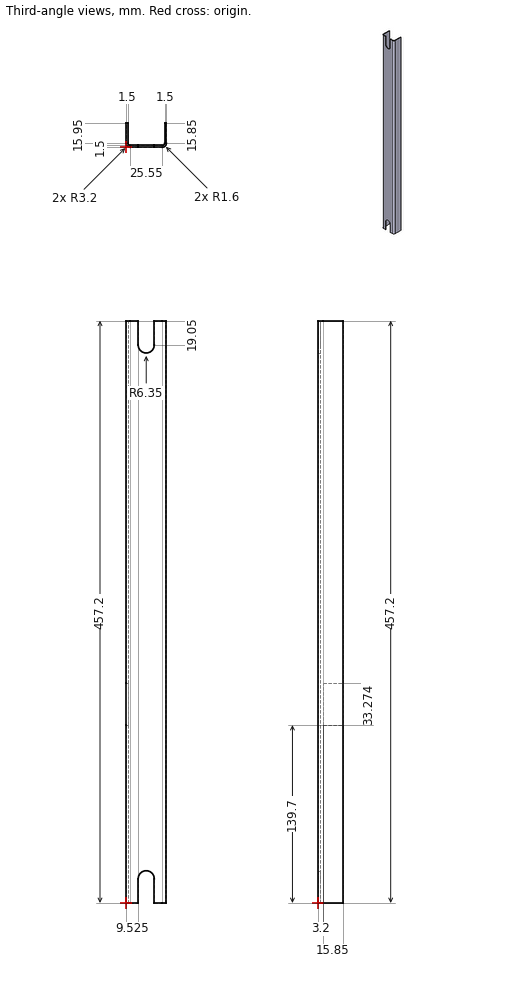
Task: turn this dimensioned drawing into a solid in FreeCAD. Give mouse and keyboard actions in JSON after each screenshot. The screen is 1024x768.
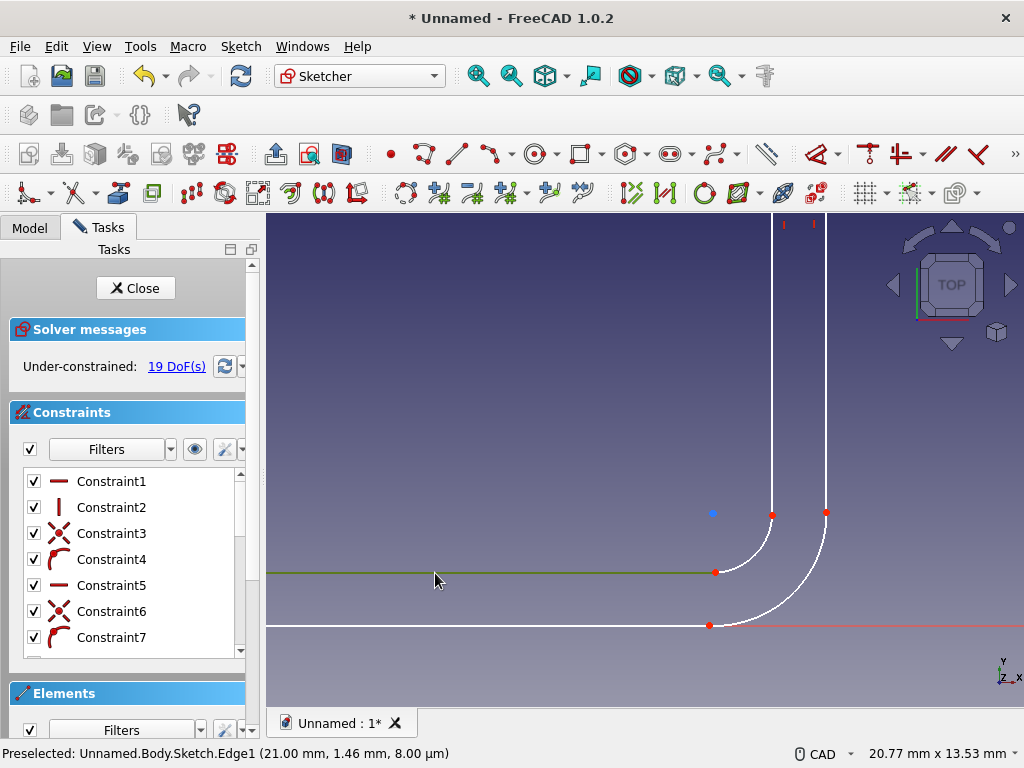
{"action": "scroll", "coordinate": [768, 566], "scroll_direction": "down", "scroll_amount": 5}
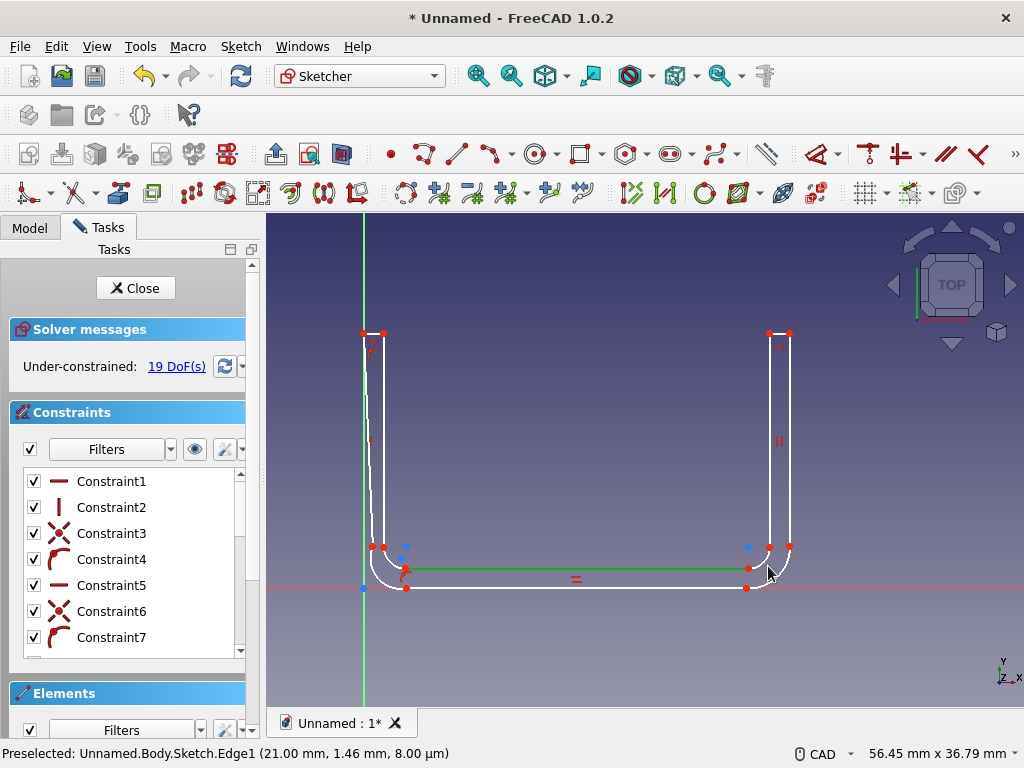
{"action": "scroll", "coordinate": [387, 557], "scroll_direction": "up", "scroll_amount": 2}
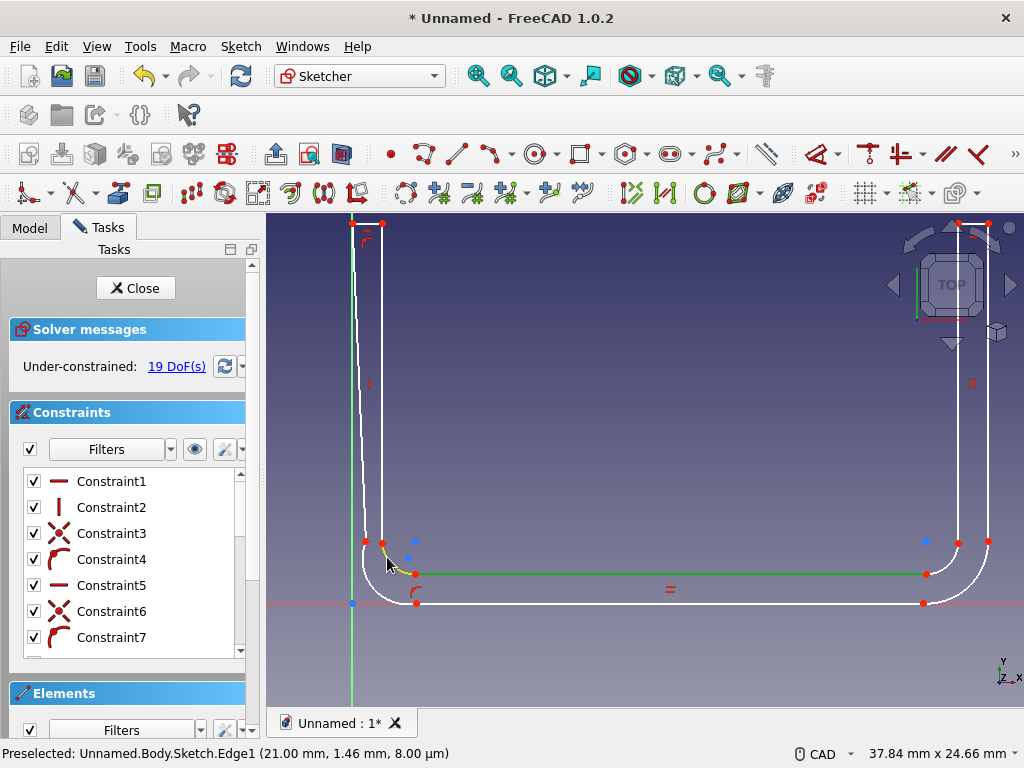
{"action": "left_click", "coordinate": [386, 557]}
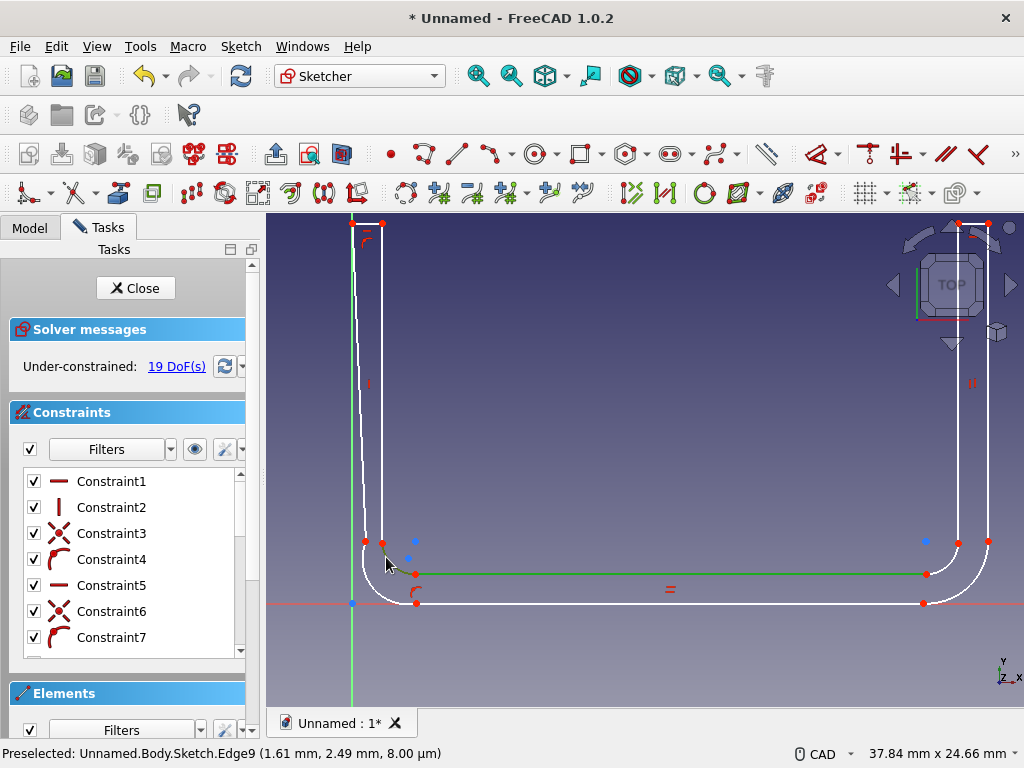
{"action": "key", "text": "t"}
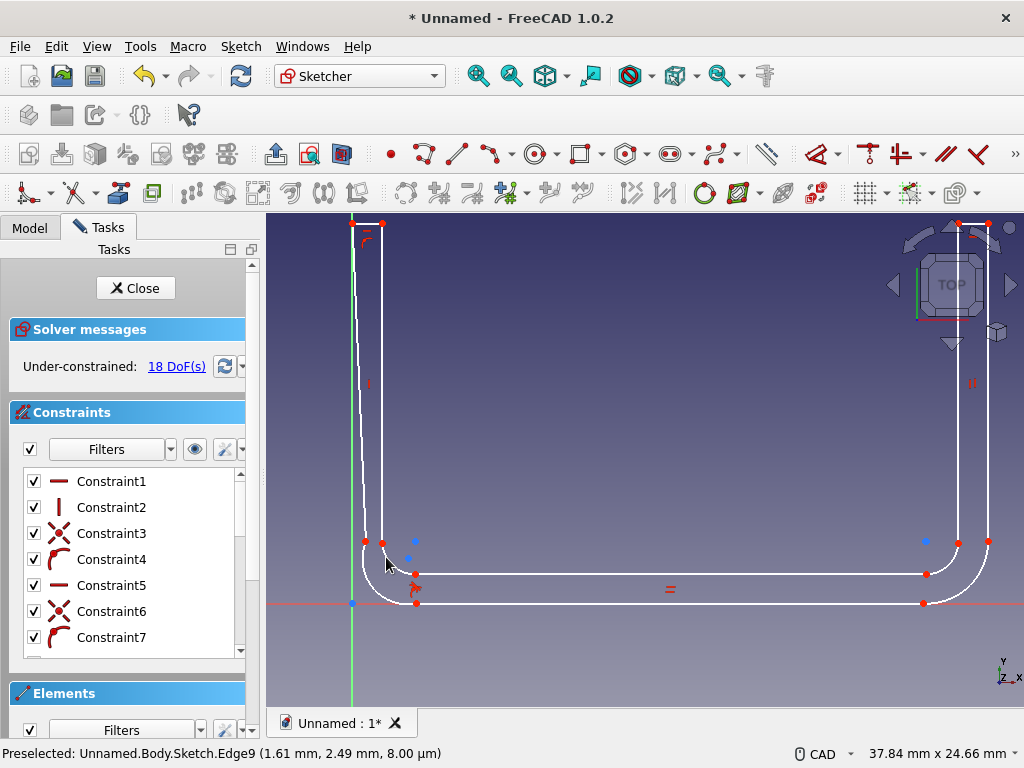
{"action": "left_click", "coordinate": [773, 574]}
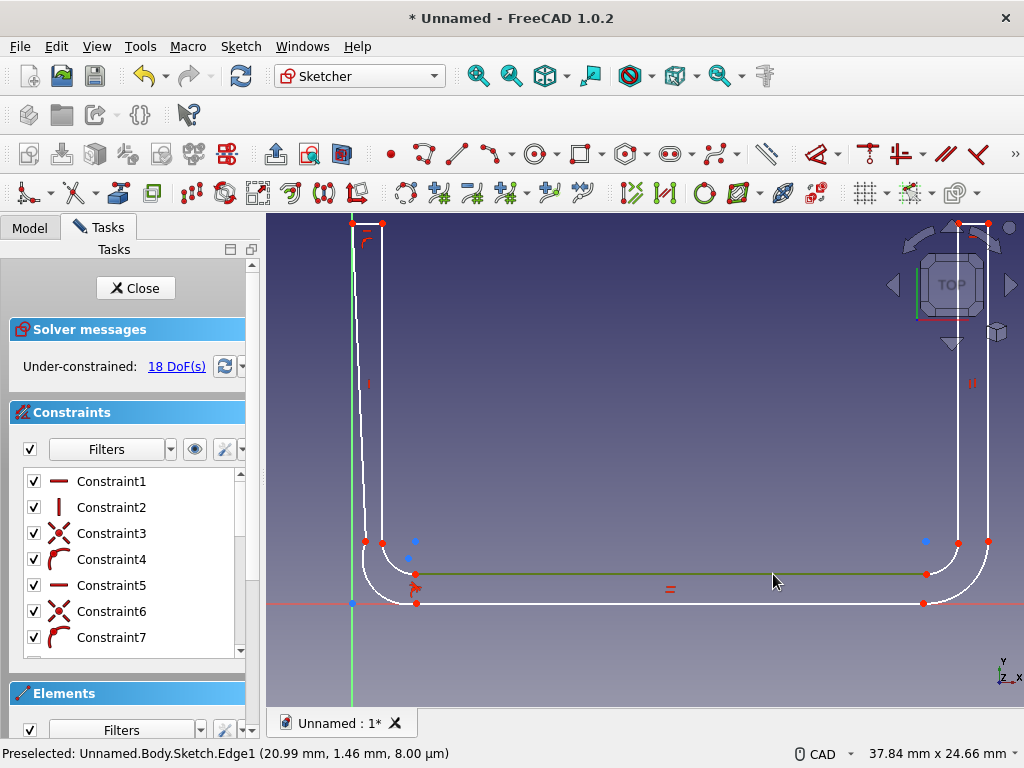
{"action": "scroll", "coordinate": [385, 556], "scroll_direction": "down", "scroll_amount": 2}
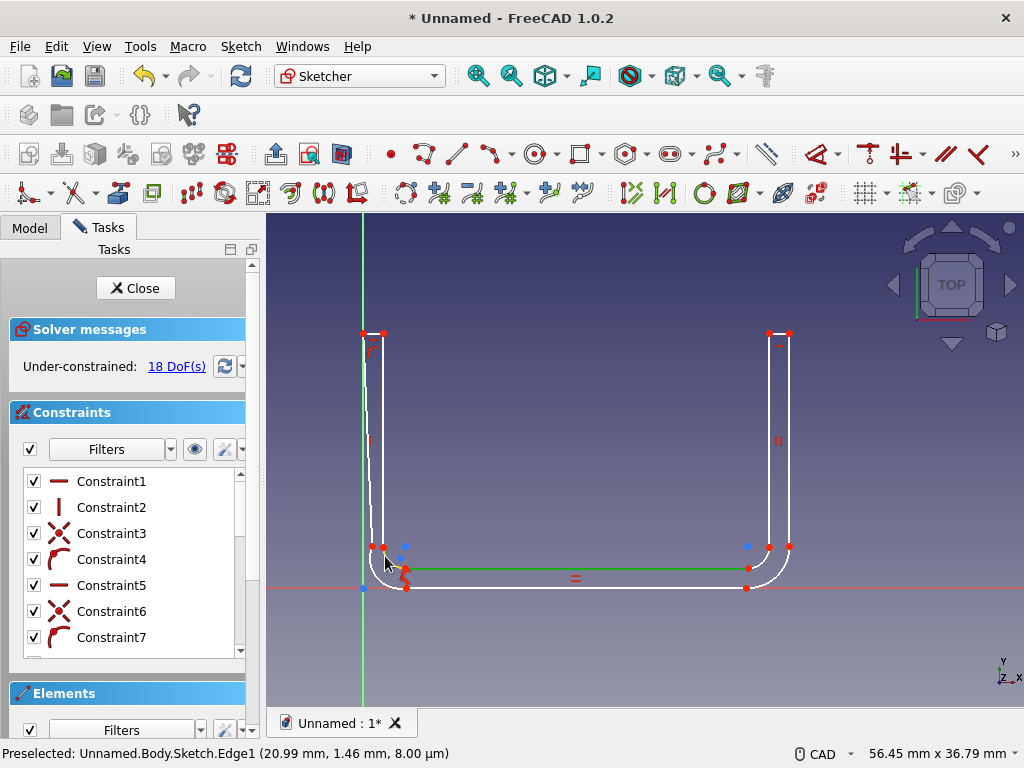
{"action": "scroll", "coordinate": [758, 566], "scroll_direction": "up", "scroll_amount": 2}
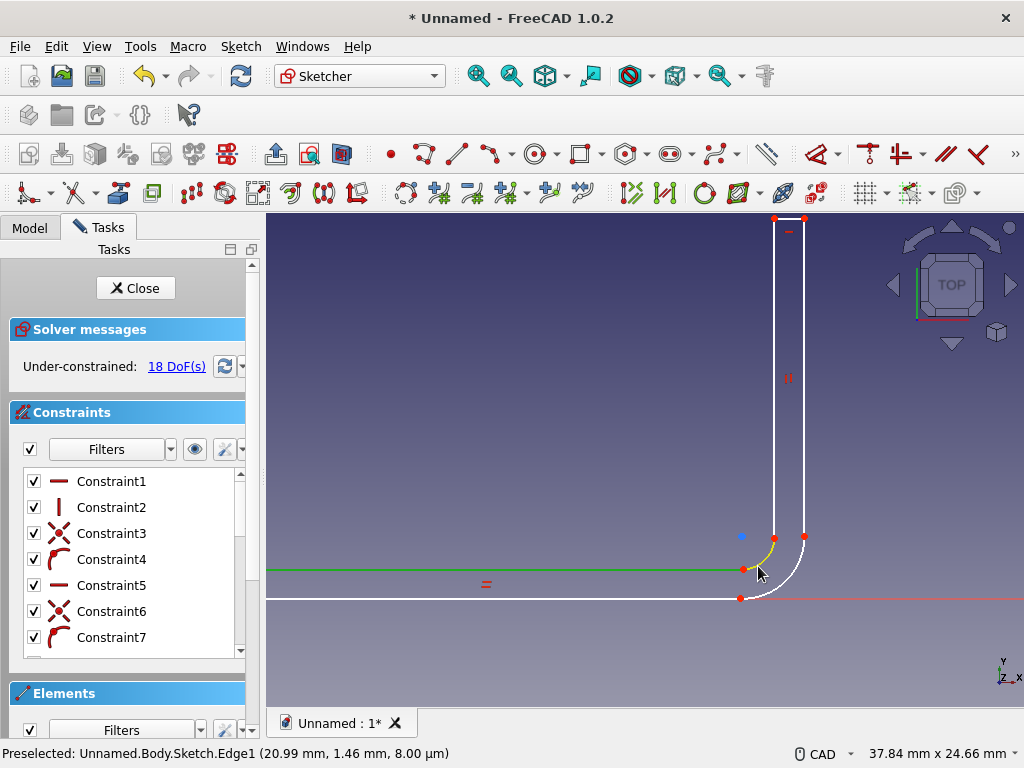
{"action": "left_click", "coordinate": [757, 566]}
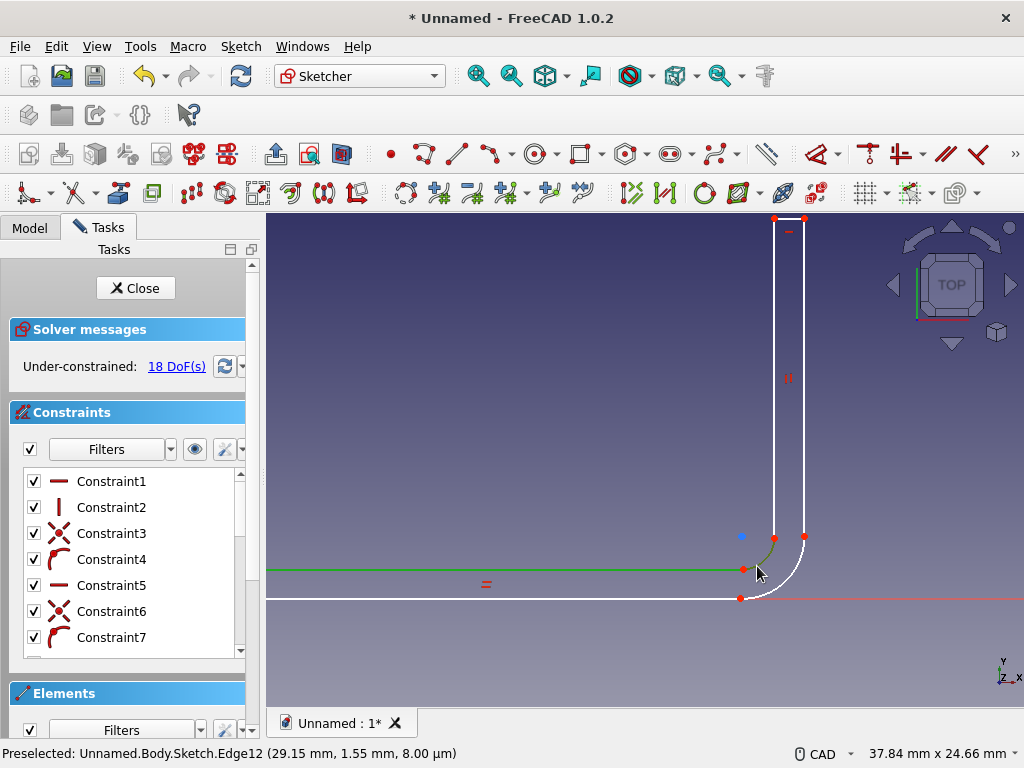
{"action": "key", "text": "t"}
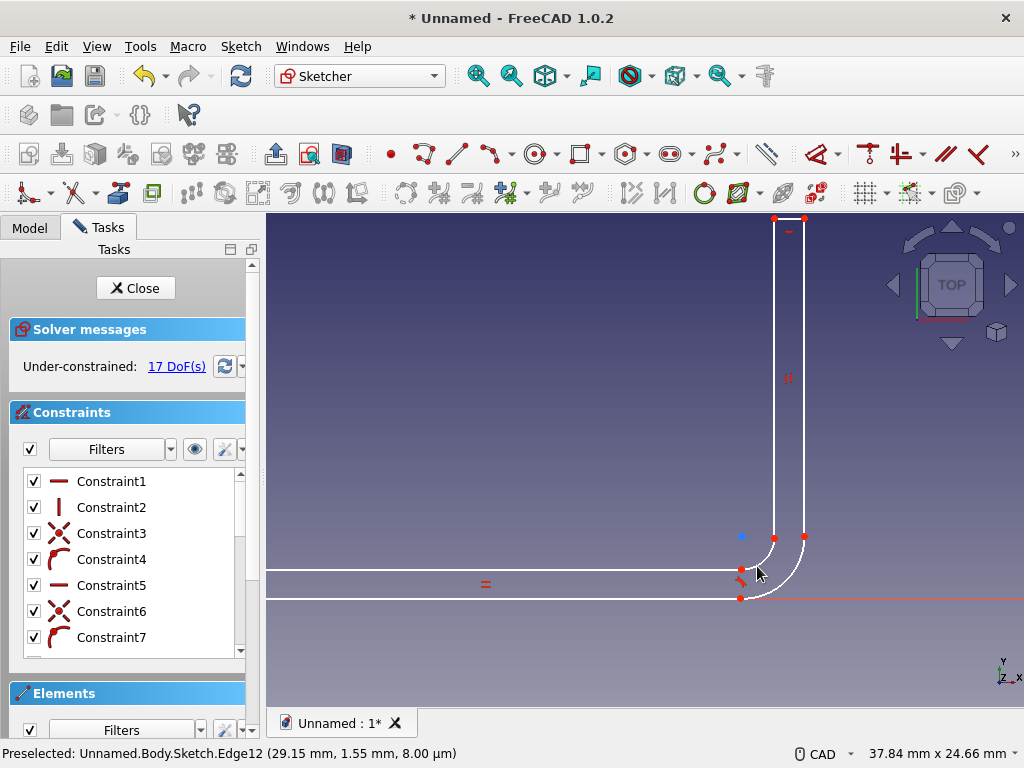
{"action": "scroll", "coordinate": [759, 566], "scroll_direction": "down", "scroll_amount": 2}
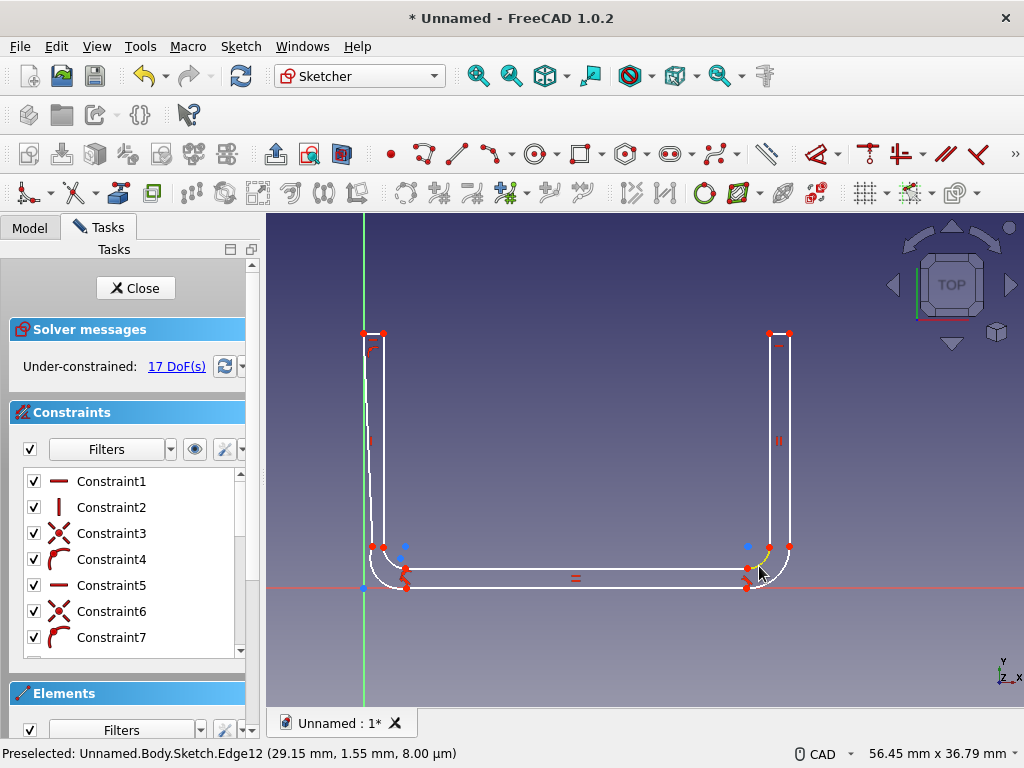
{"action": "left_click", "coordinate": [384, 483]}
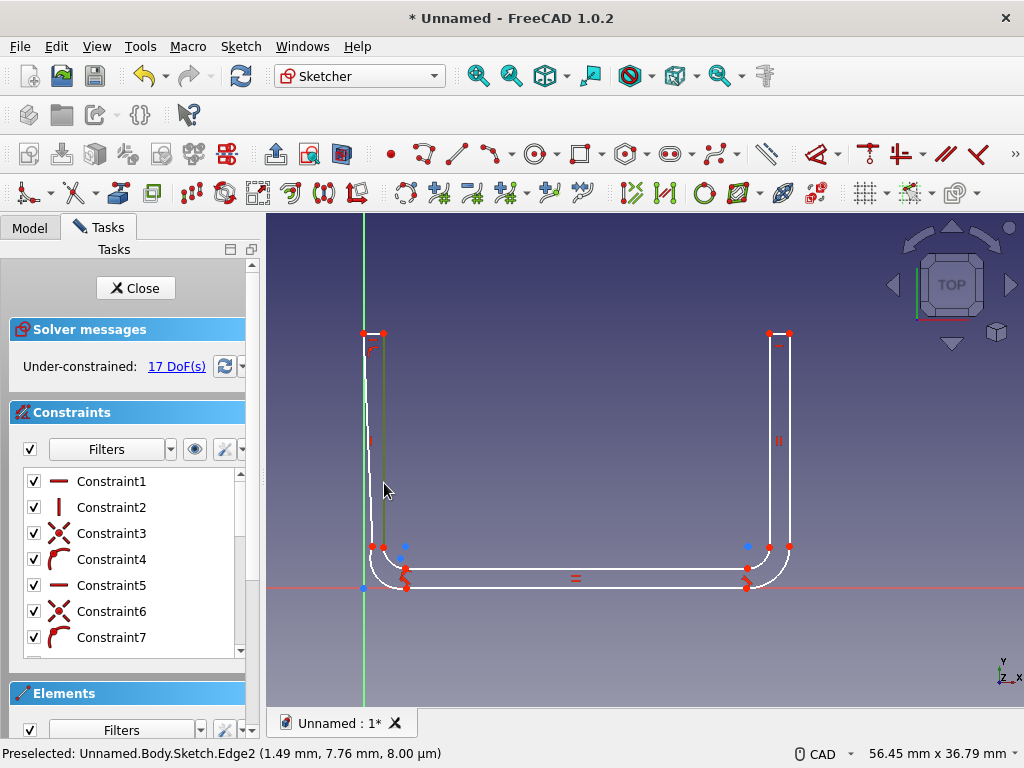
{"action": "scroll", "coordinate": [386, 557], "scroll_direction": "up", "scroll_amount": 2}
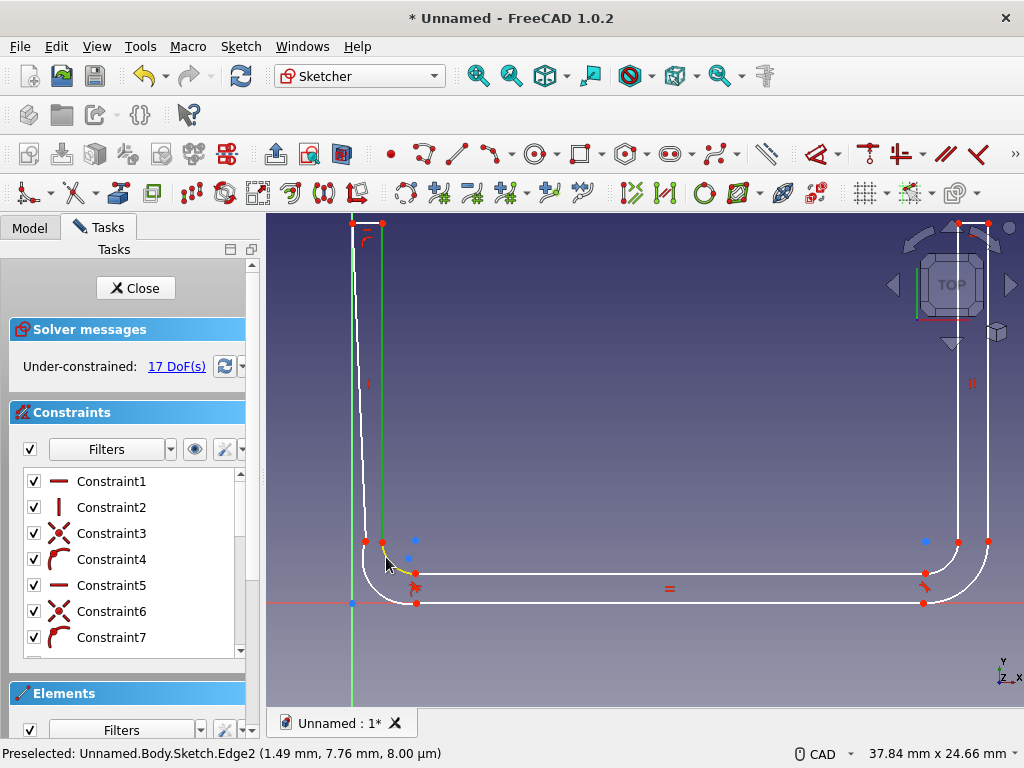
{"action": "left_click", "coordinate": [387, 557]}